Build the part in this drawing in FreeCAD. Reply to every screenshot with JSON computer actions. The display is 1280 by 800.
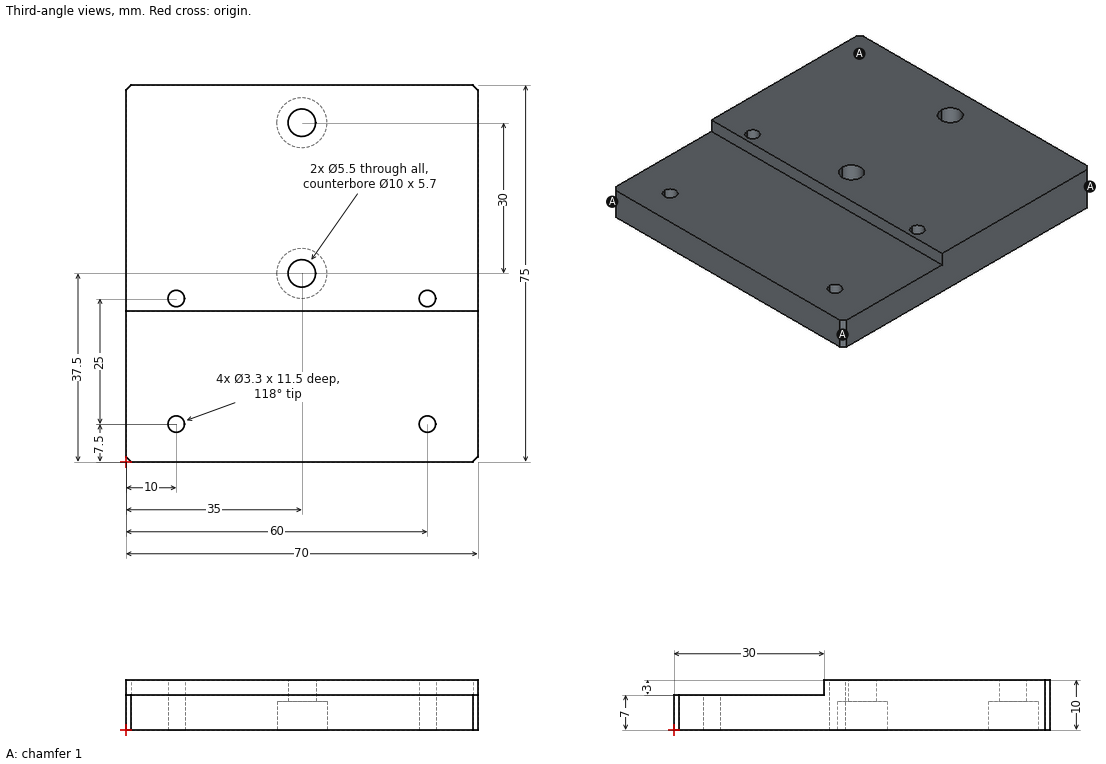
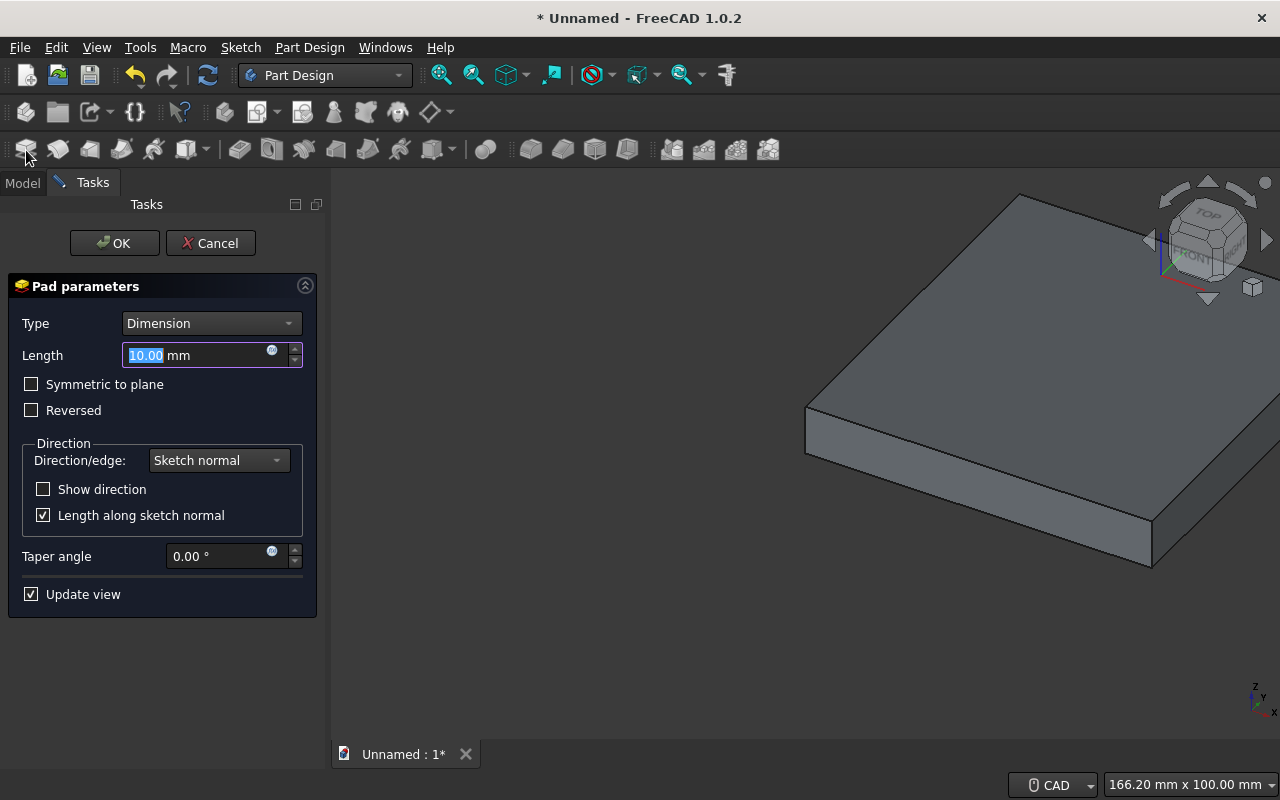
{"action": "type", "text": "10"}
{"action": "key", "text": "Tab"}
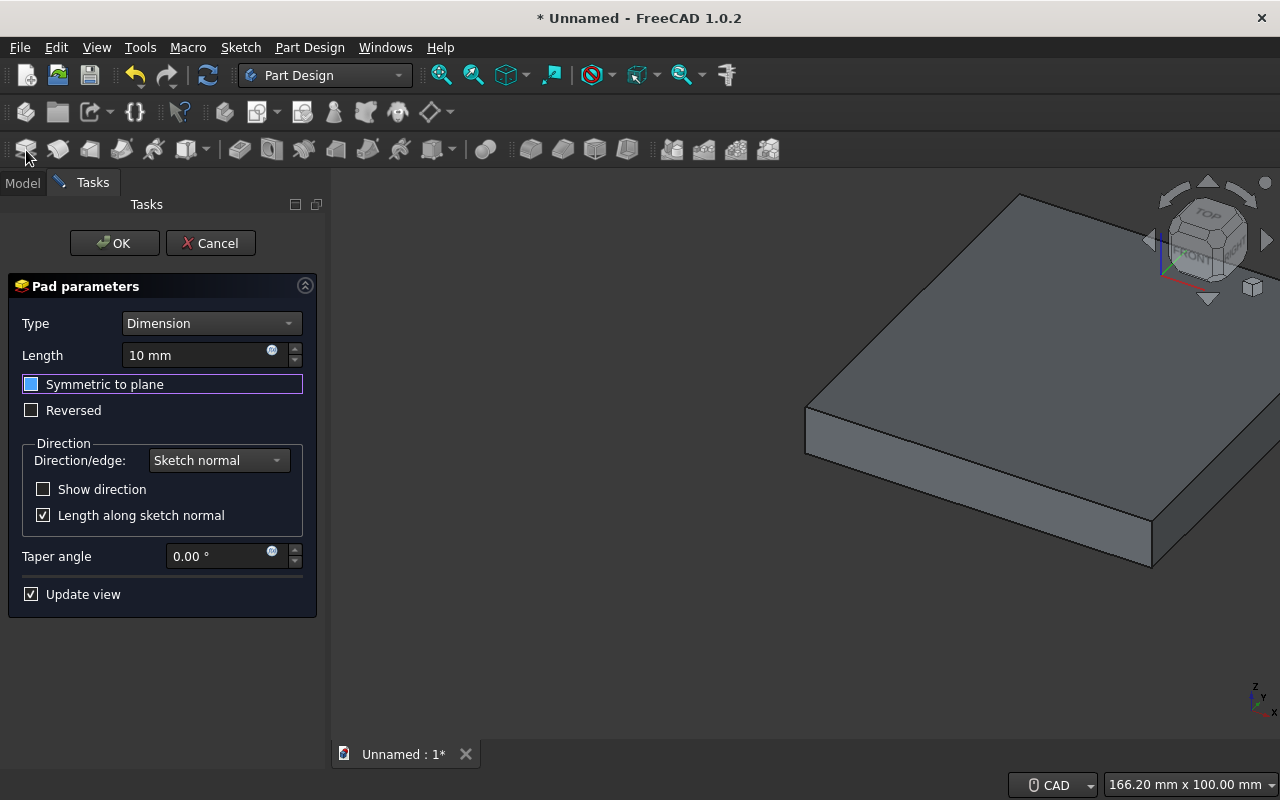
{"action": "left_click", "coordinate": [115, 243]}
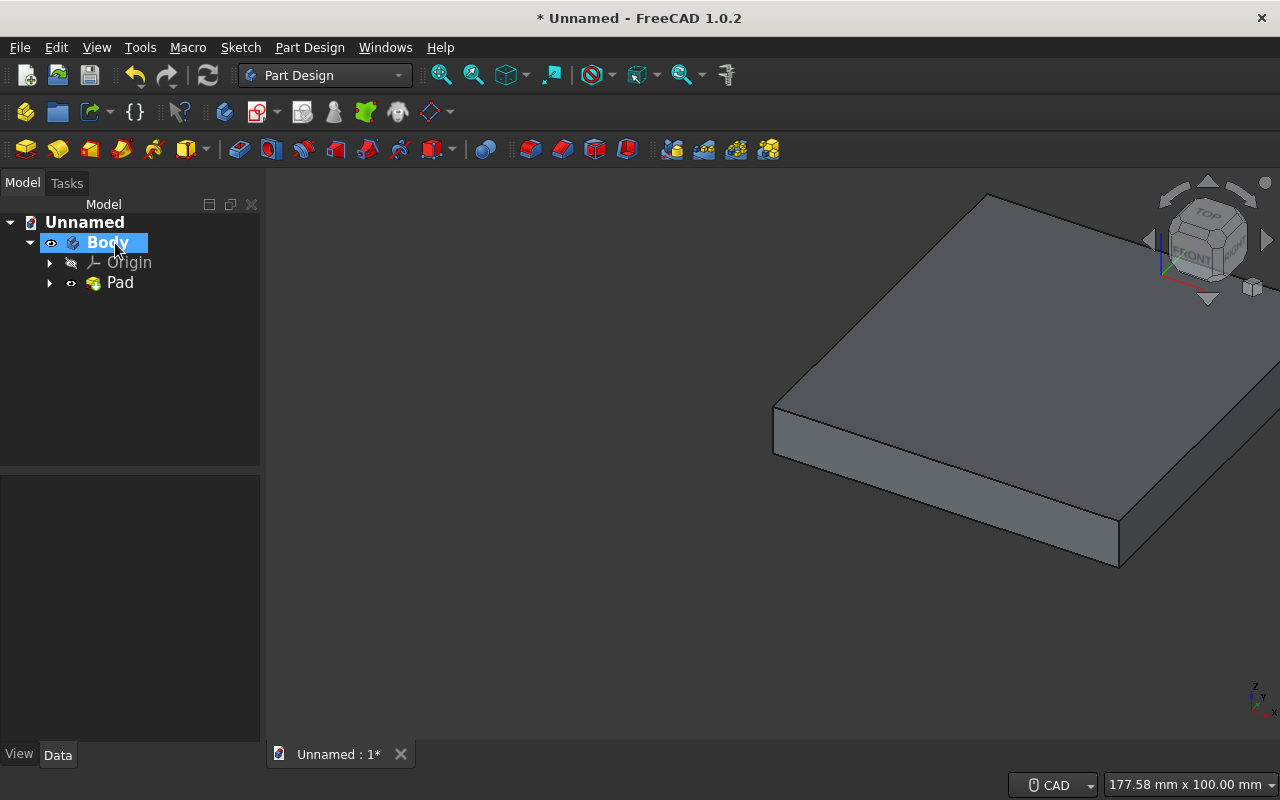
{"action": "left_click", "coordinate": [442, 76]}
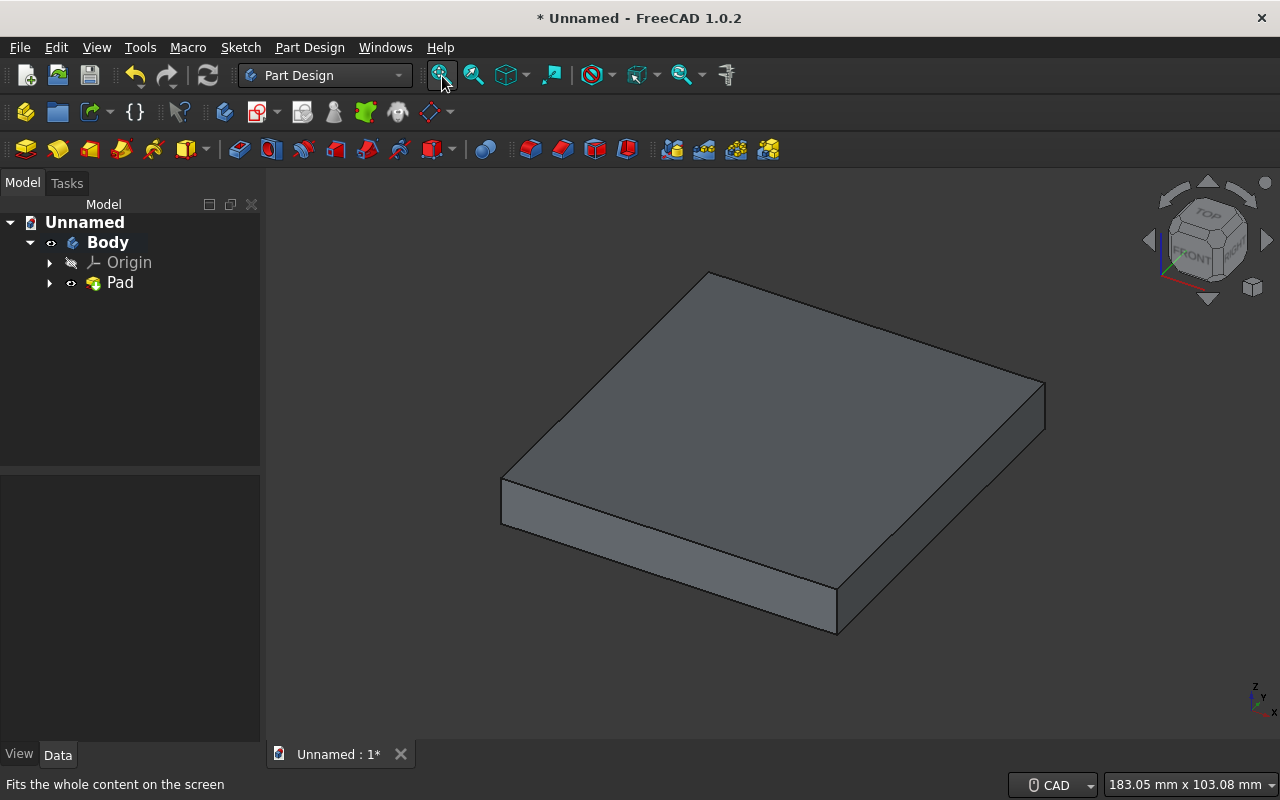
{"action": "key", "text": "6"}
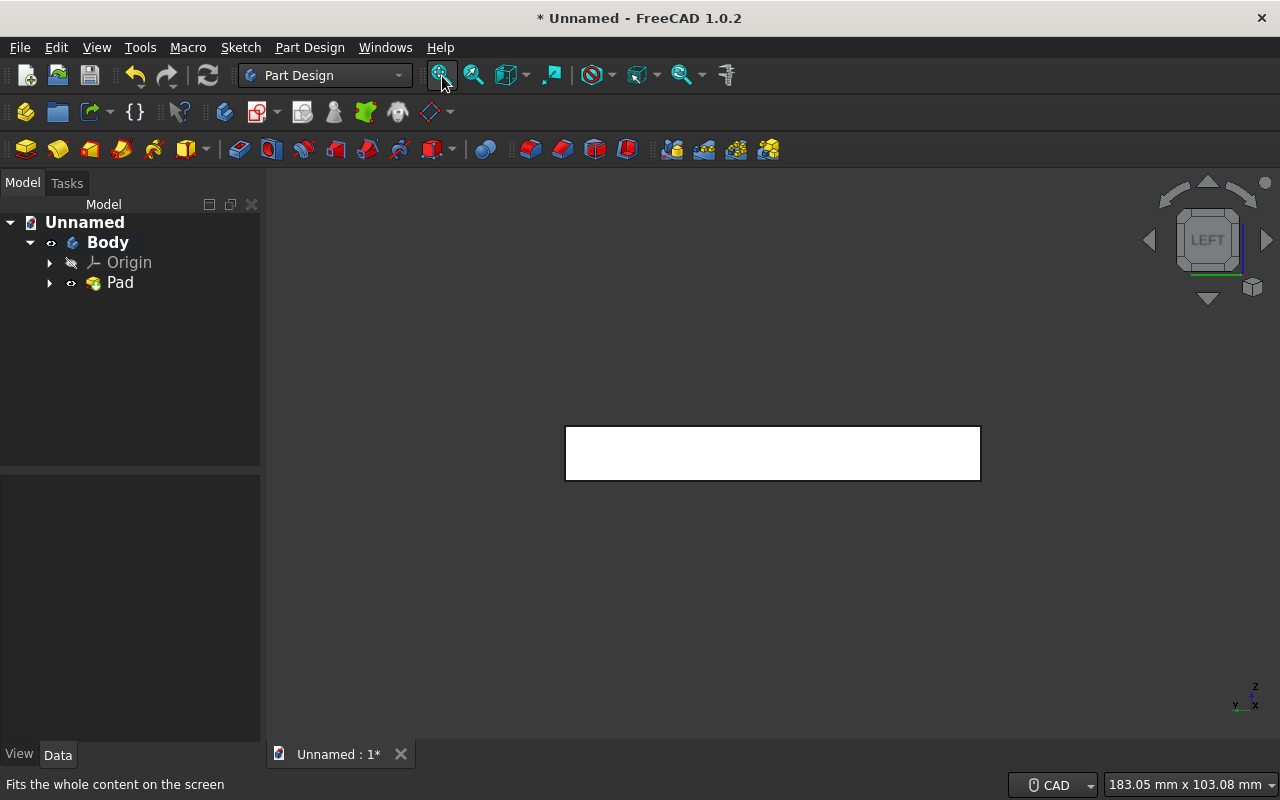
{"action": "left_click", "coordinate": [442, 76]}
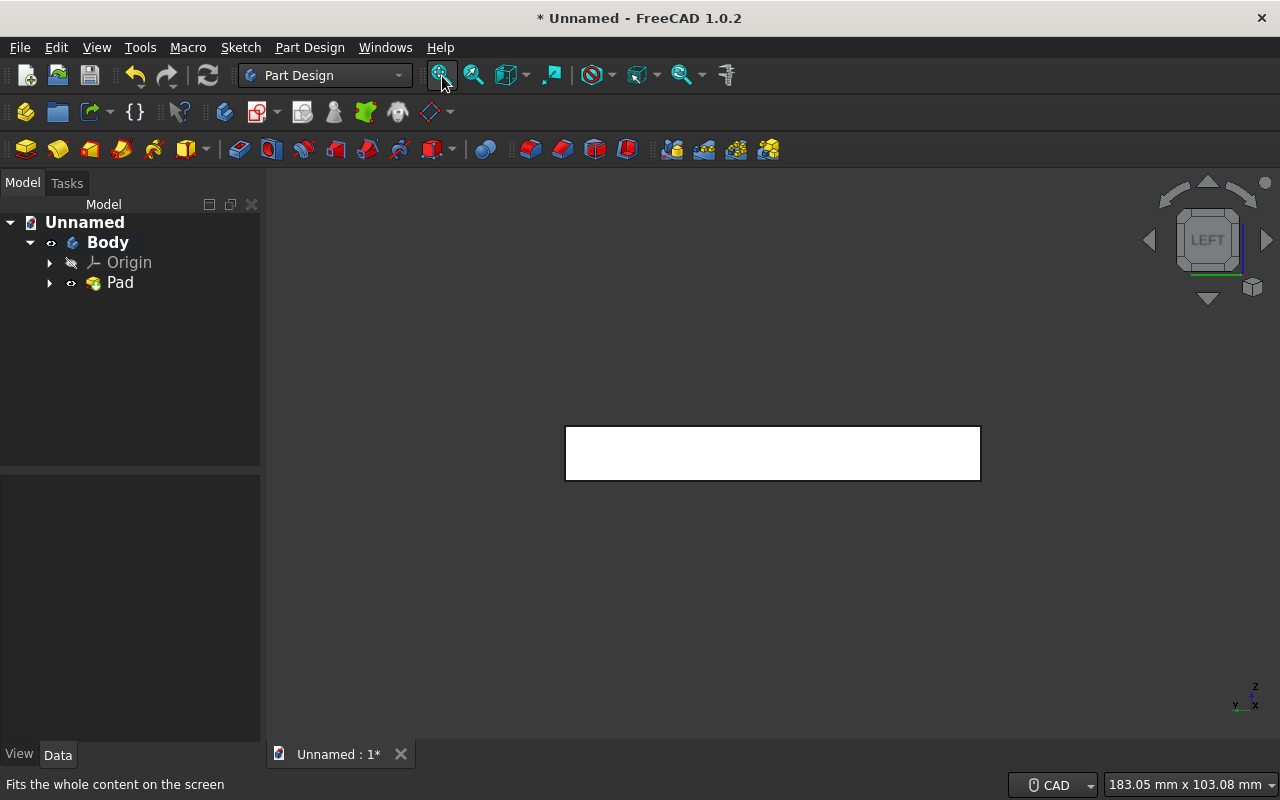
{"action": "left_click", "coordinate": [595, 452]}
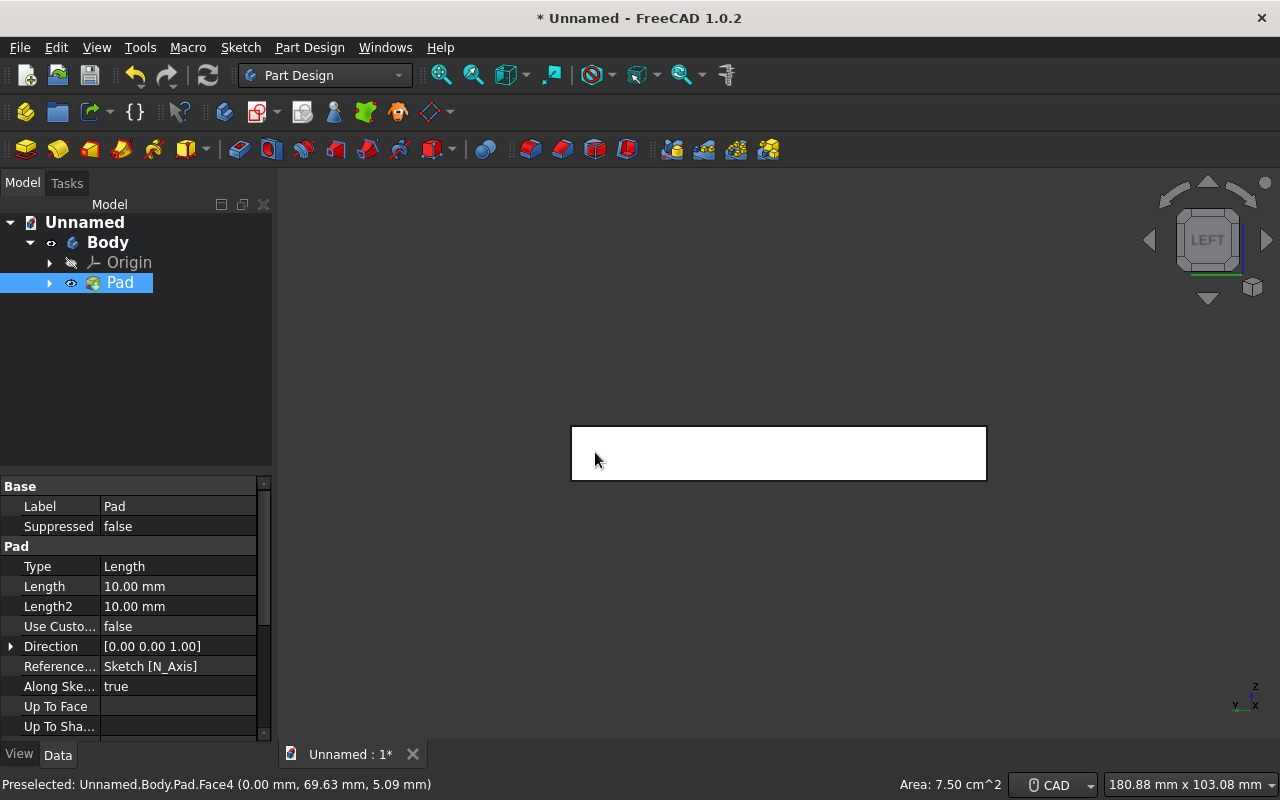
{"action": "left_click", "coordinate": [258, 112]}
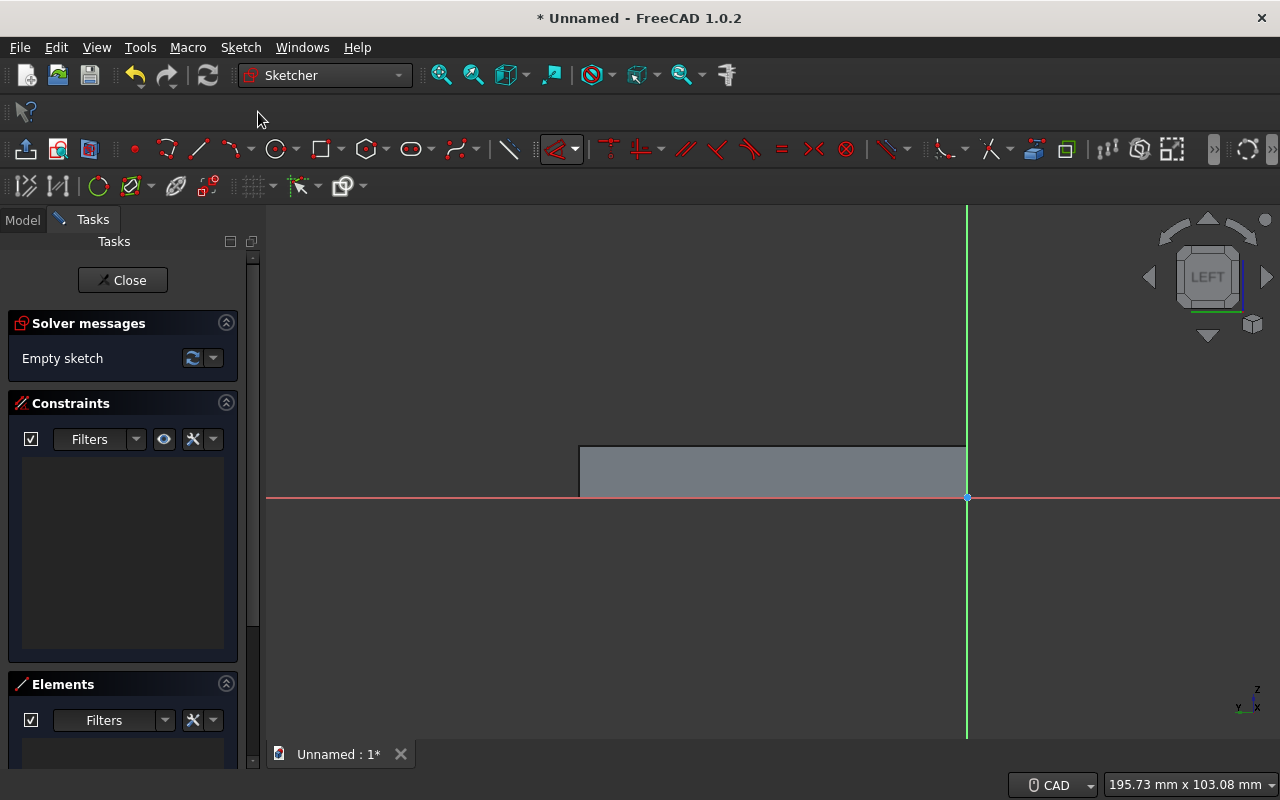
{"action": "scroll", "coordinate": [950, 472], "scroll_direction": "up", "scroll_amount": 7}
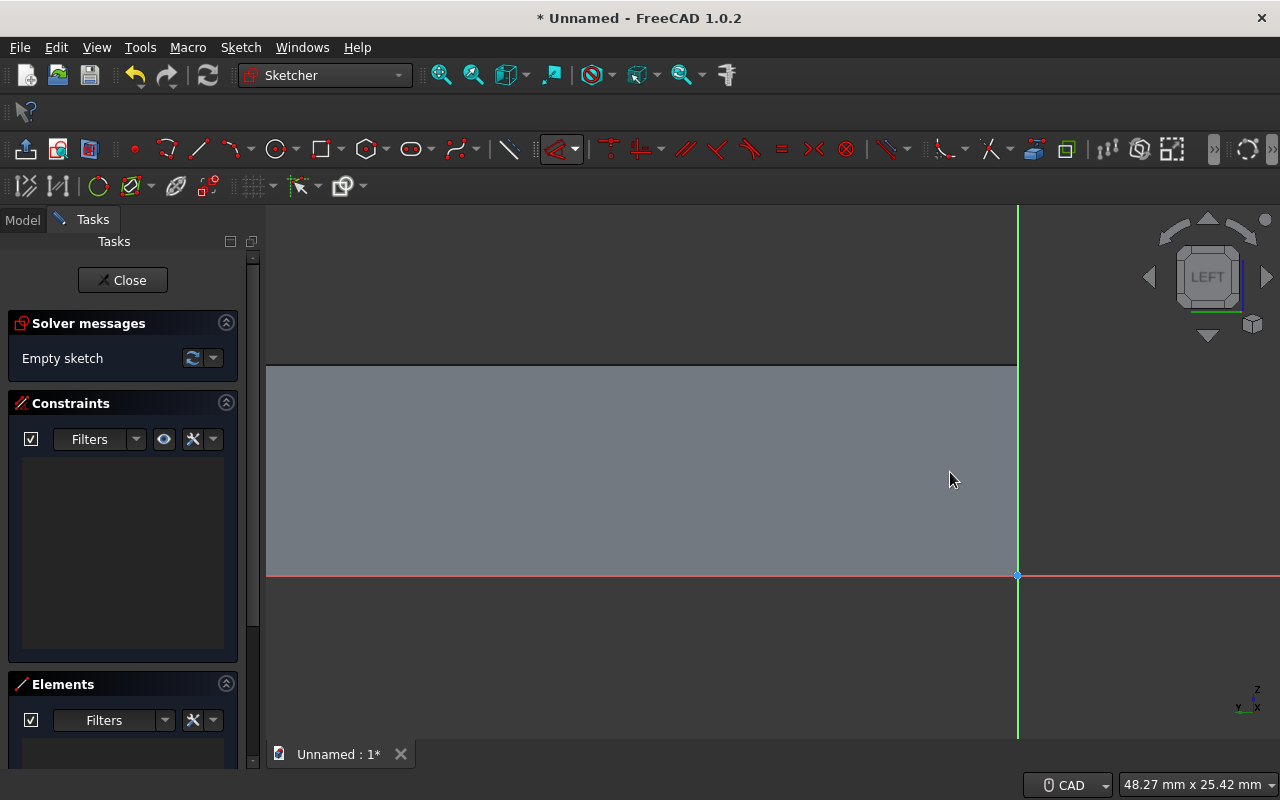
{"action": "left_click", "coordinate": [322, 150]}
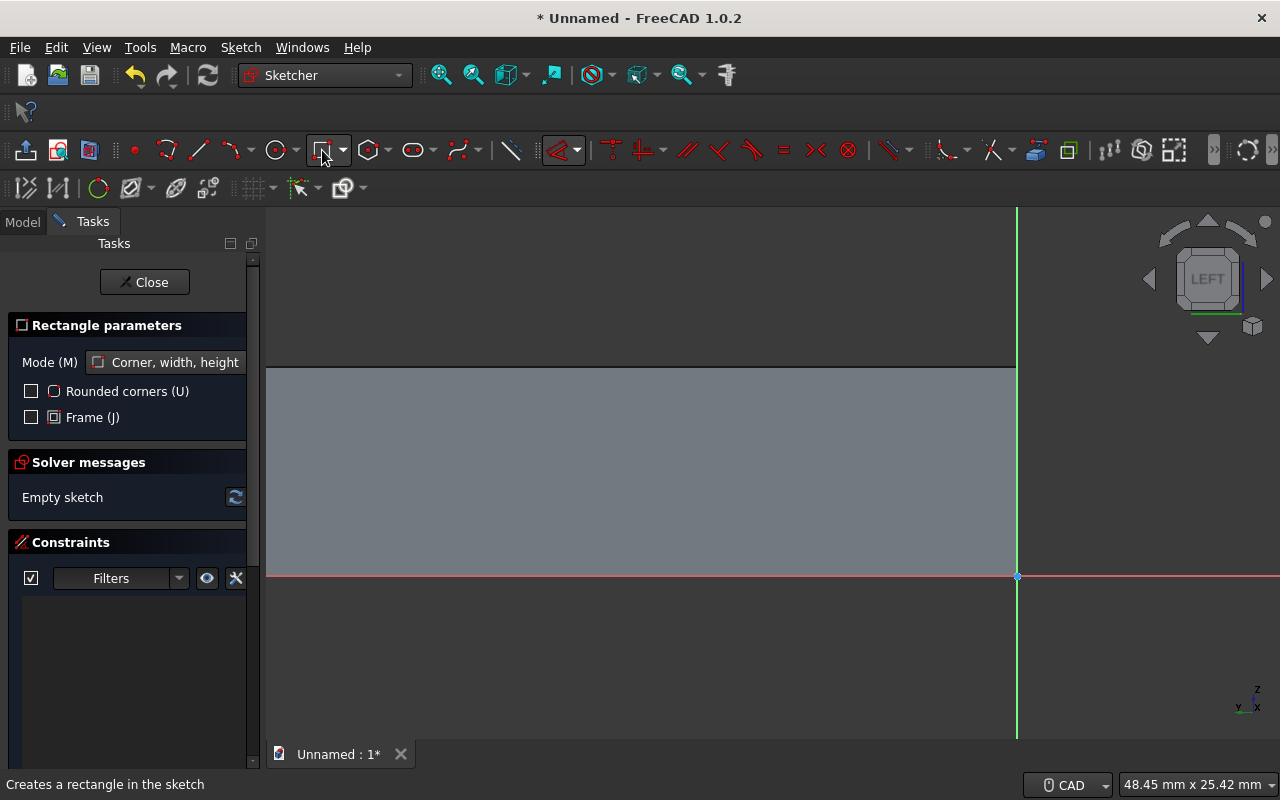
{"action": "left_click", "coordinate": [389, 367]}
{"action": "left_click", "coordinate": [1017, 430]}
{"action": "key", "text": "Escape"}